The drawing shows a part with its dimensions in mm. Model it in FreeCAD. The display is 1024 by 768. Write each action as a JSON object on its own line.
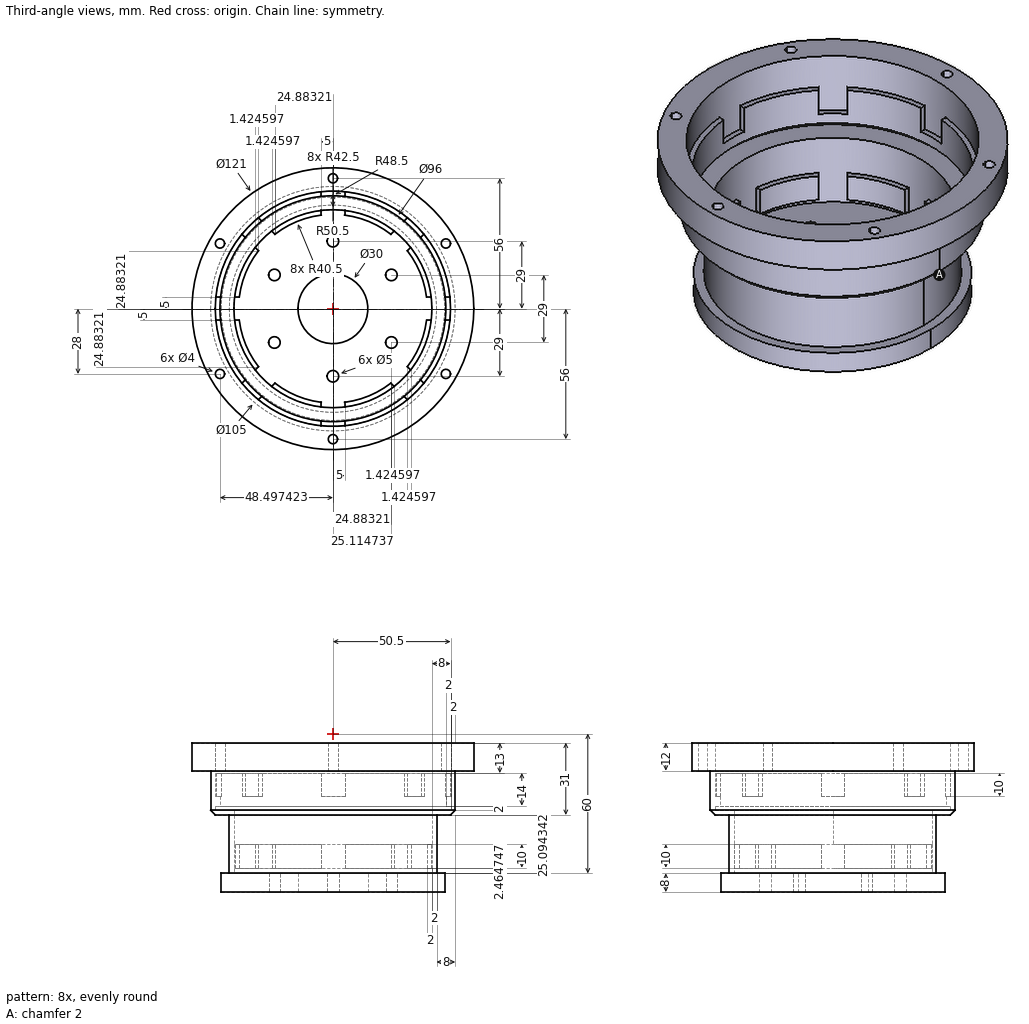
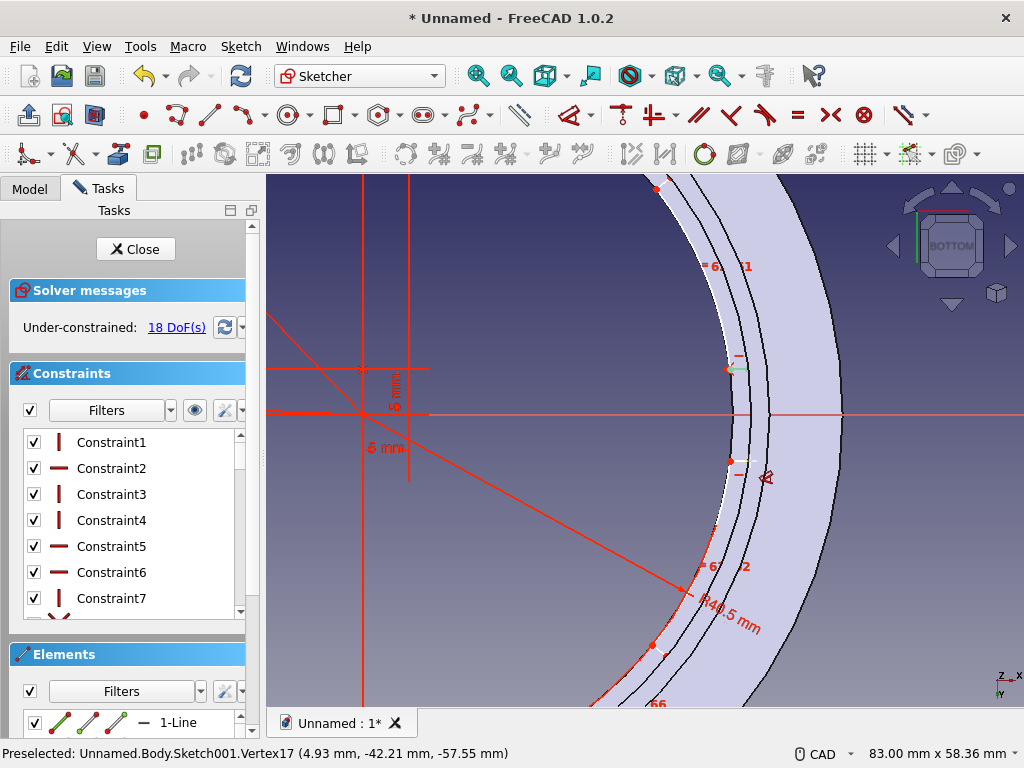
{"action": "left_click", "coordinate": [749, 461]}
{"action": "left_click", "coordinate": [783, 438]}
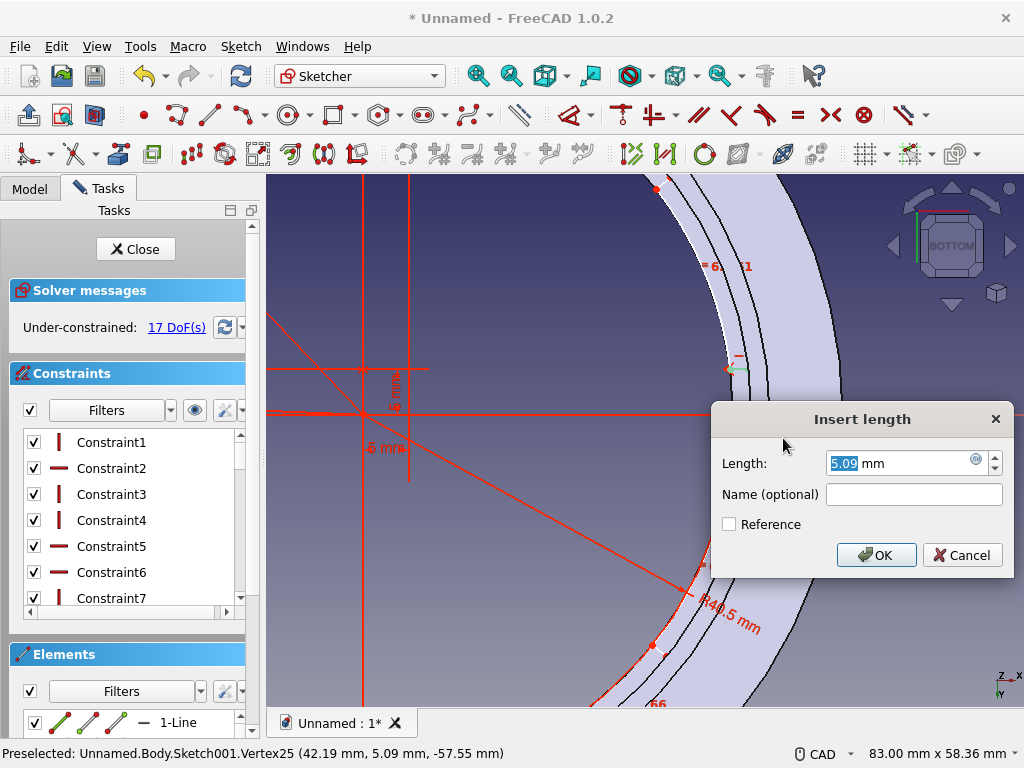
{"action": "type", "text": "5"}
{"action": "key", "text": "Return"}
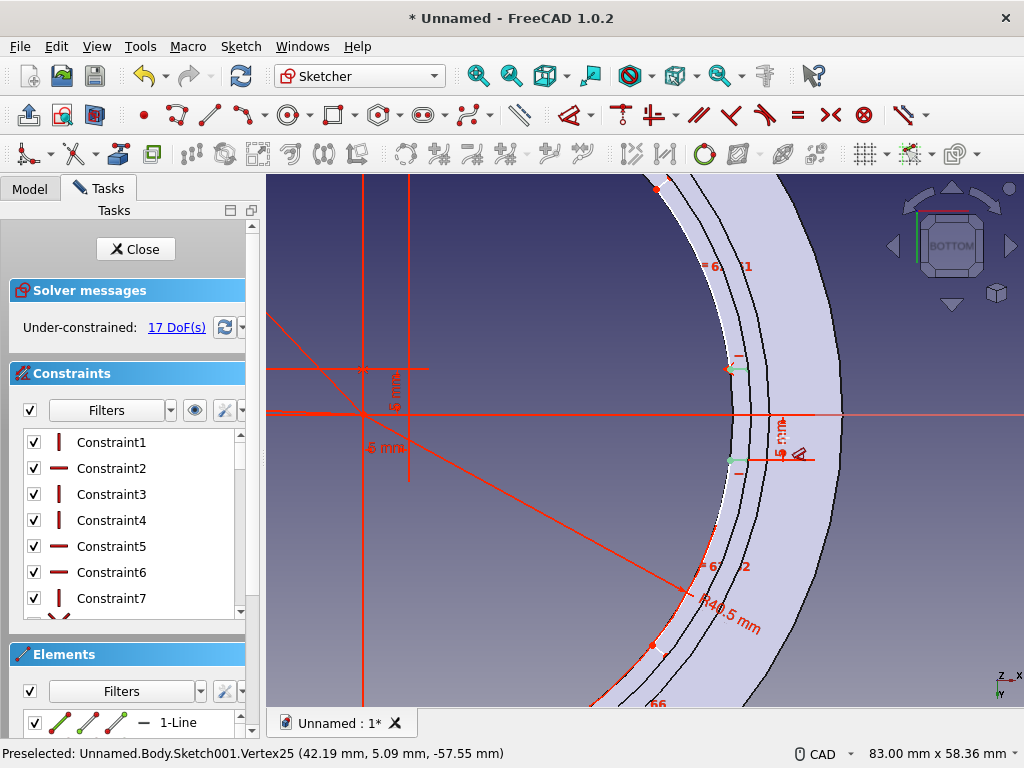
{"action": "scroll", "coordinate": [751, 461], "scroll_direction": "down", "scroll_amount": 4}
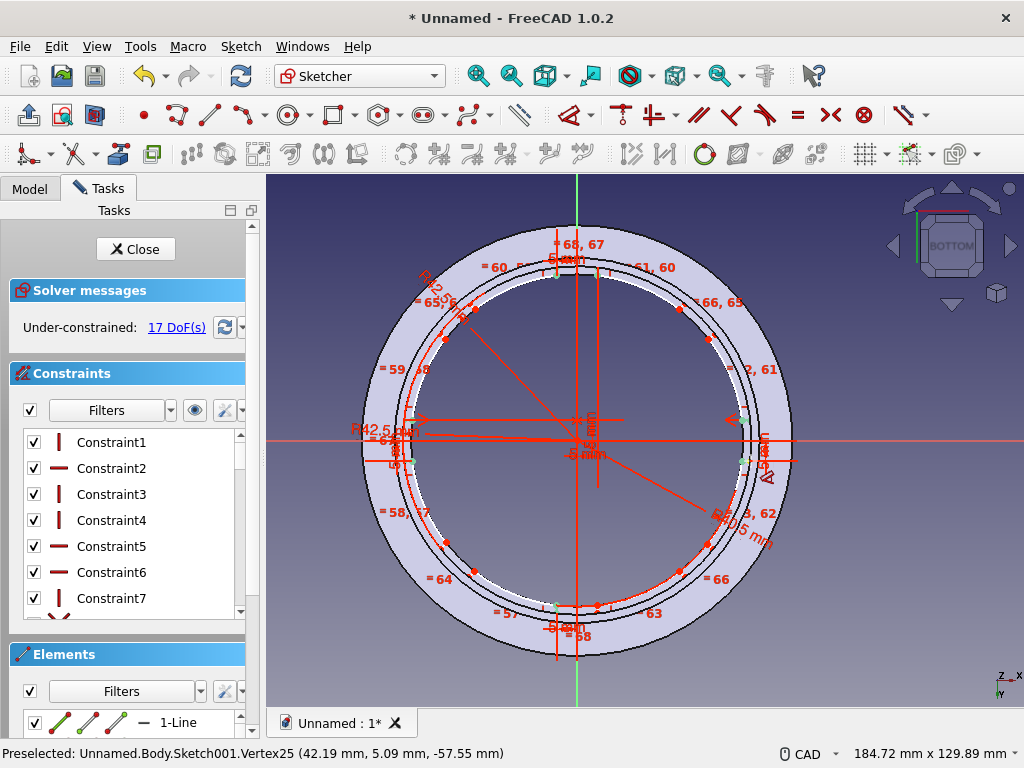
{"action": "scroll", "coordinate": [598, 605], "scroll_direction": "up", "scroll_amount": 4}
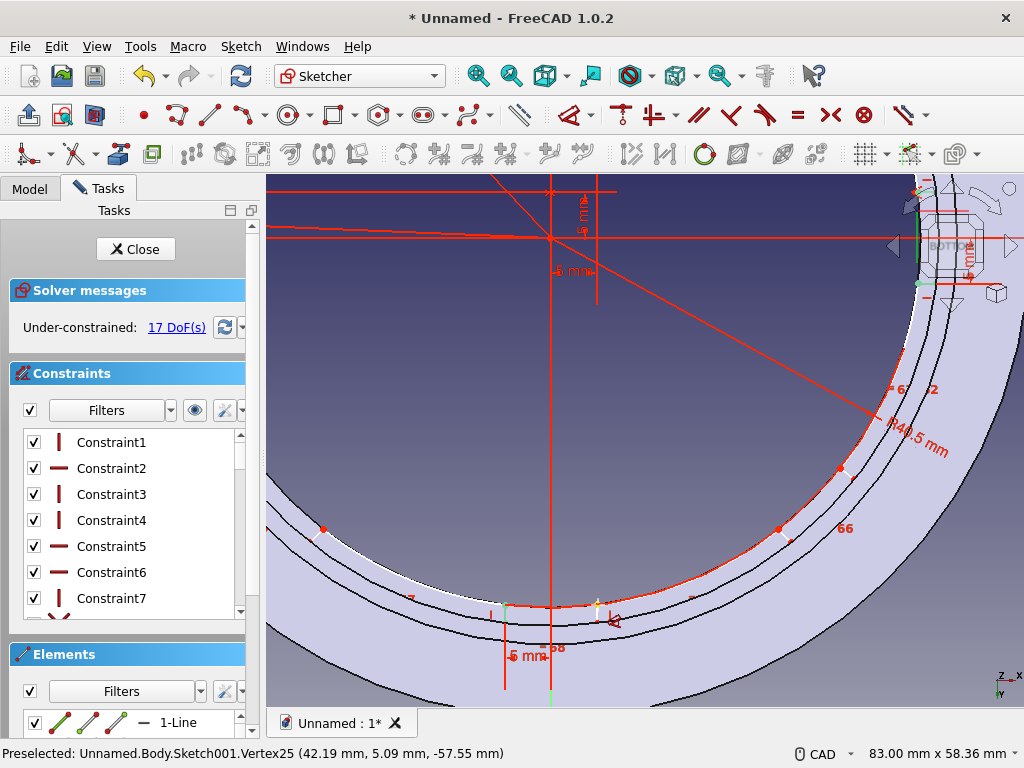
{"action": "left_click", "coordinate": [597, 605]}
{"action": "left_click", "coordinate": [574, 639]}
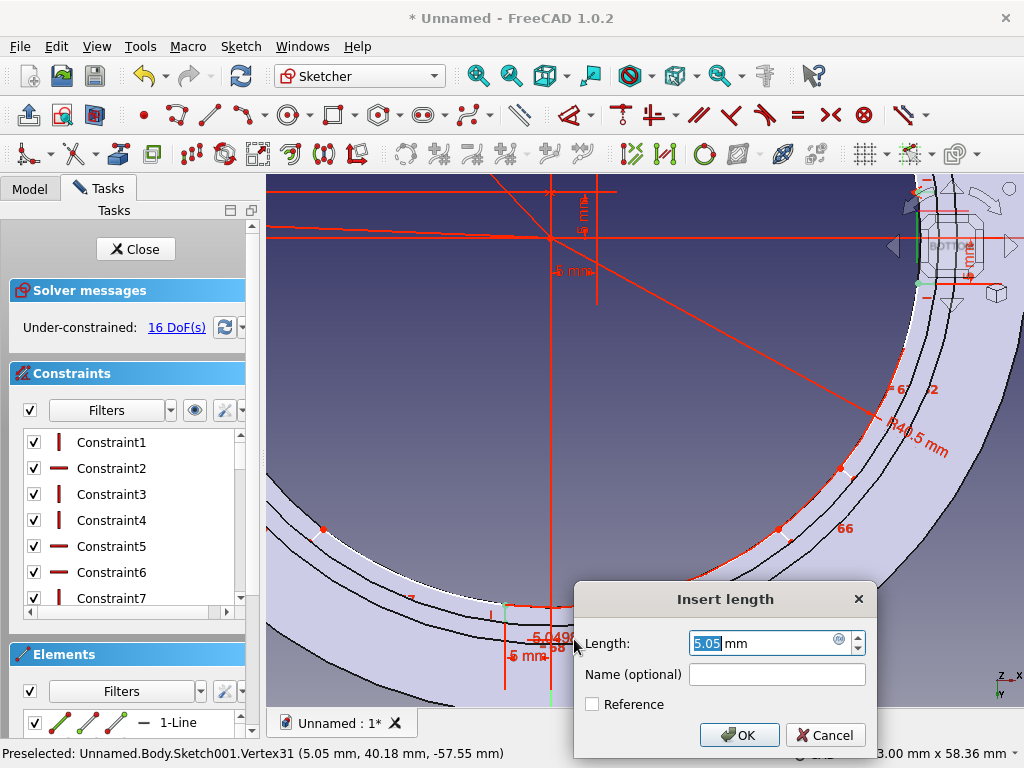
{"action": "type", "text": "5"}
{"action": "key", "text": "Return"}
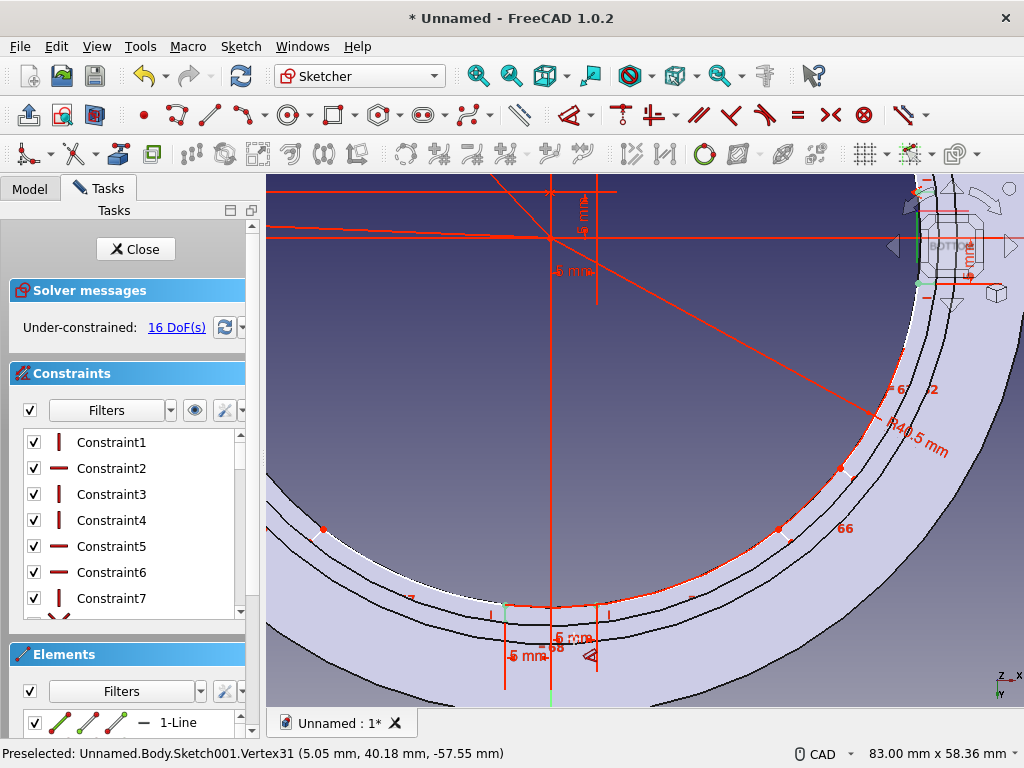
{"action": "left_click", "coordinate": [323, 530]}
{"action": "left_click", "coordinate": [437, 564]}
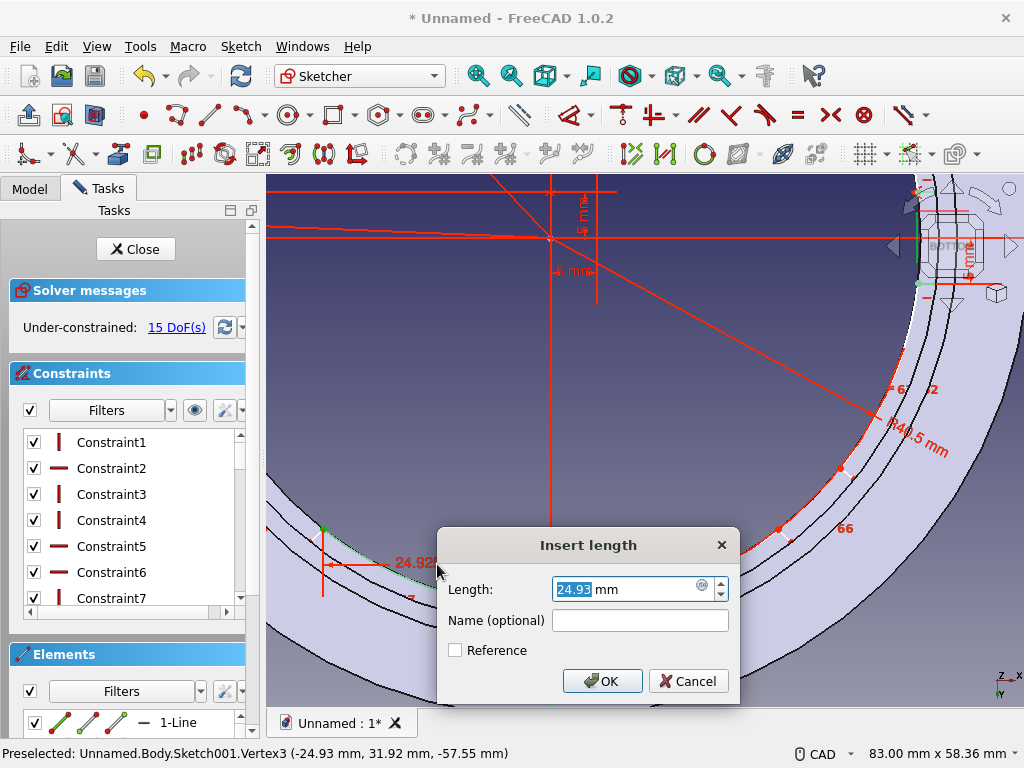
{"action": "type", "text": "24.88321"}
{"action": "key", "text": "Return"}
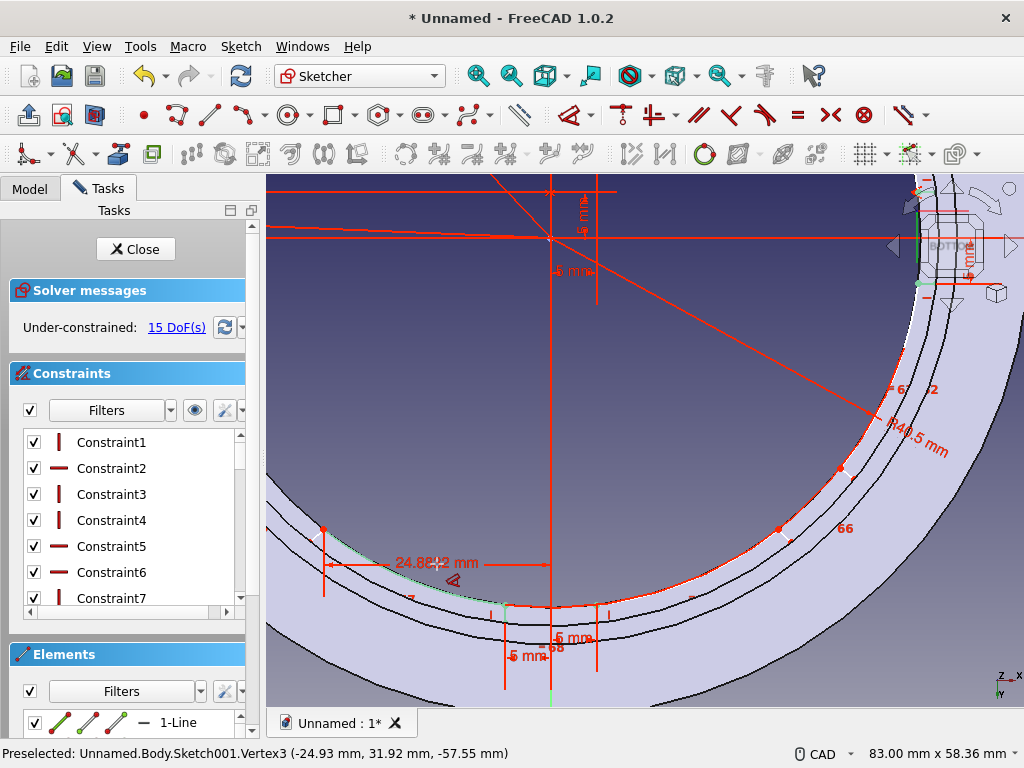
{"action": "scroll", "coordinate": [597, 606], "scroll_direction": "down", "scroll_amount": 4}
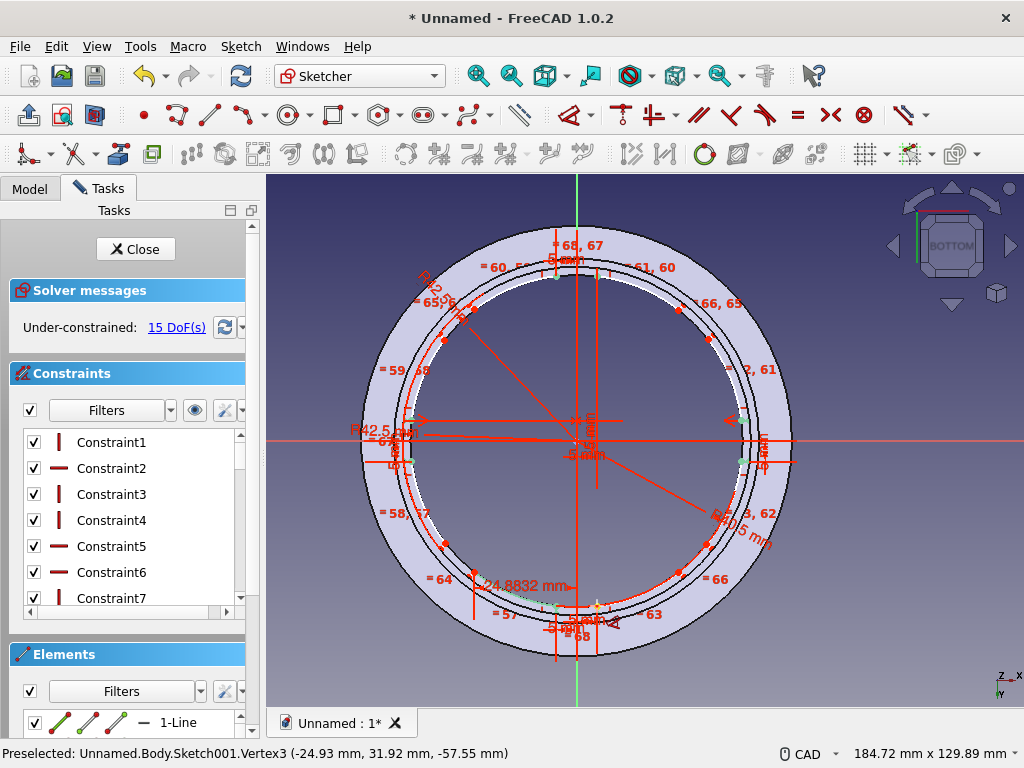
{"action": "scroll", "coordinate": [446, 544], "scroll_direction": "up", "scroll_amount": 2}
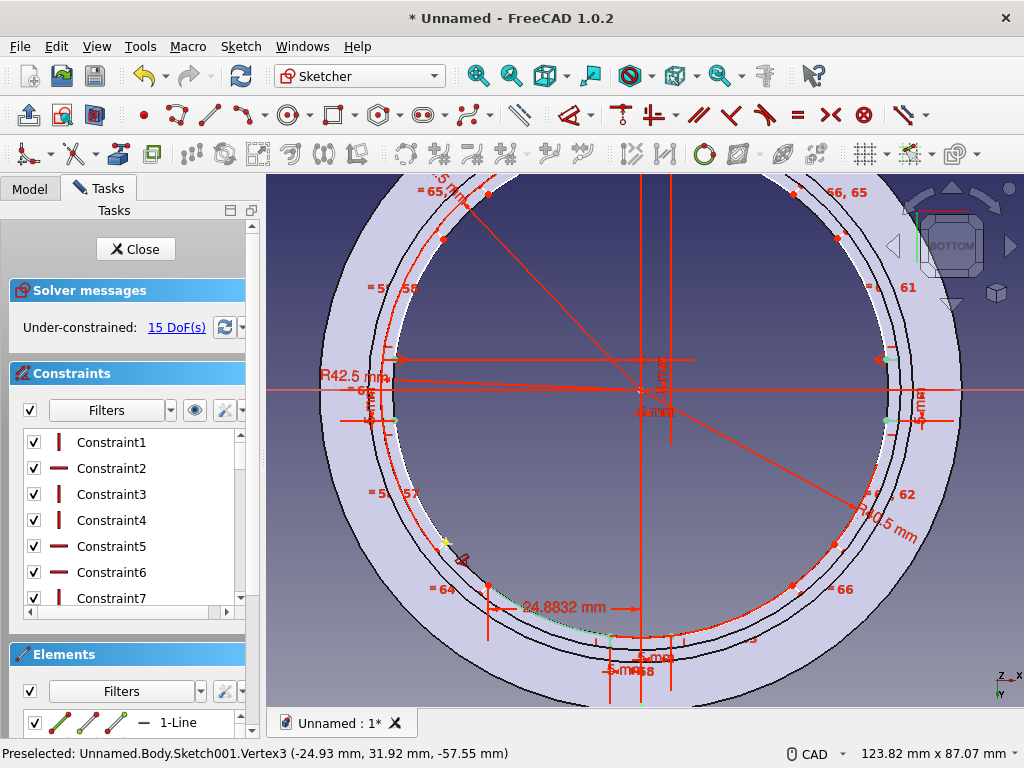
{"action": "left_click", "coordinate": [445, 543]}
{"action": "left_click", "coordinate": [411, 431]}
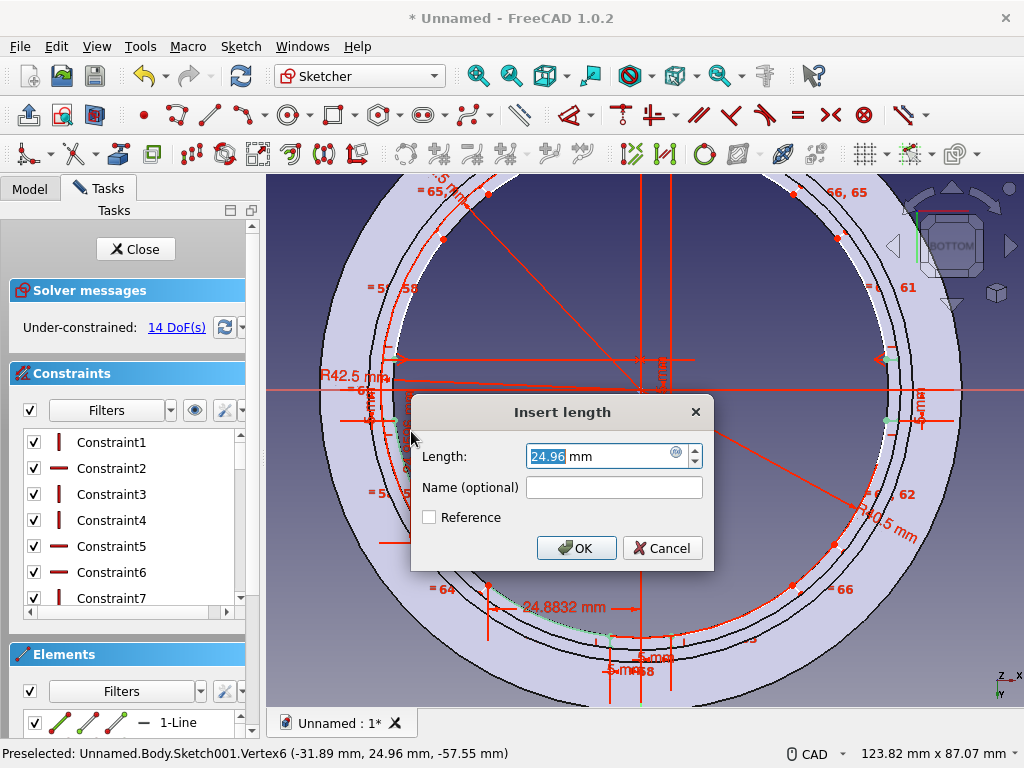
{"action": "type", "text": "24.88321"}
{"action": "key", "text": "Return"}